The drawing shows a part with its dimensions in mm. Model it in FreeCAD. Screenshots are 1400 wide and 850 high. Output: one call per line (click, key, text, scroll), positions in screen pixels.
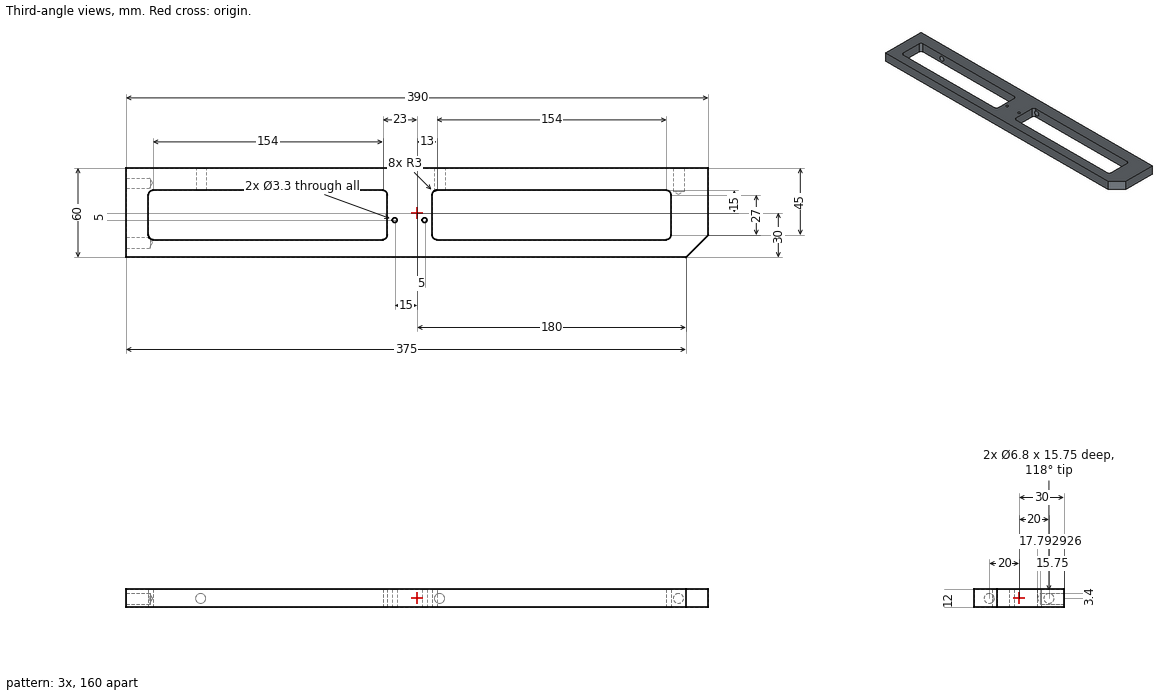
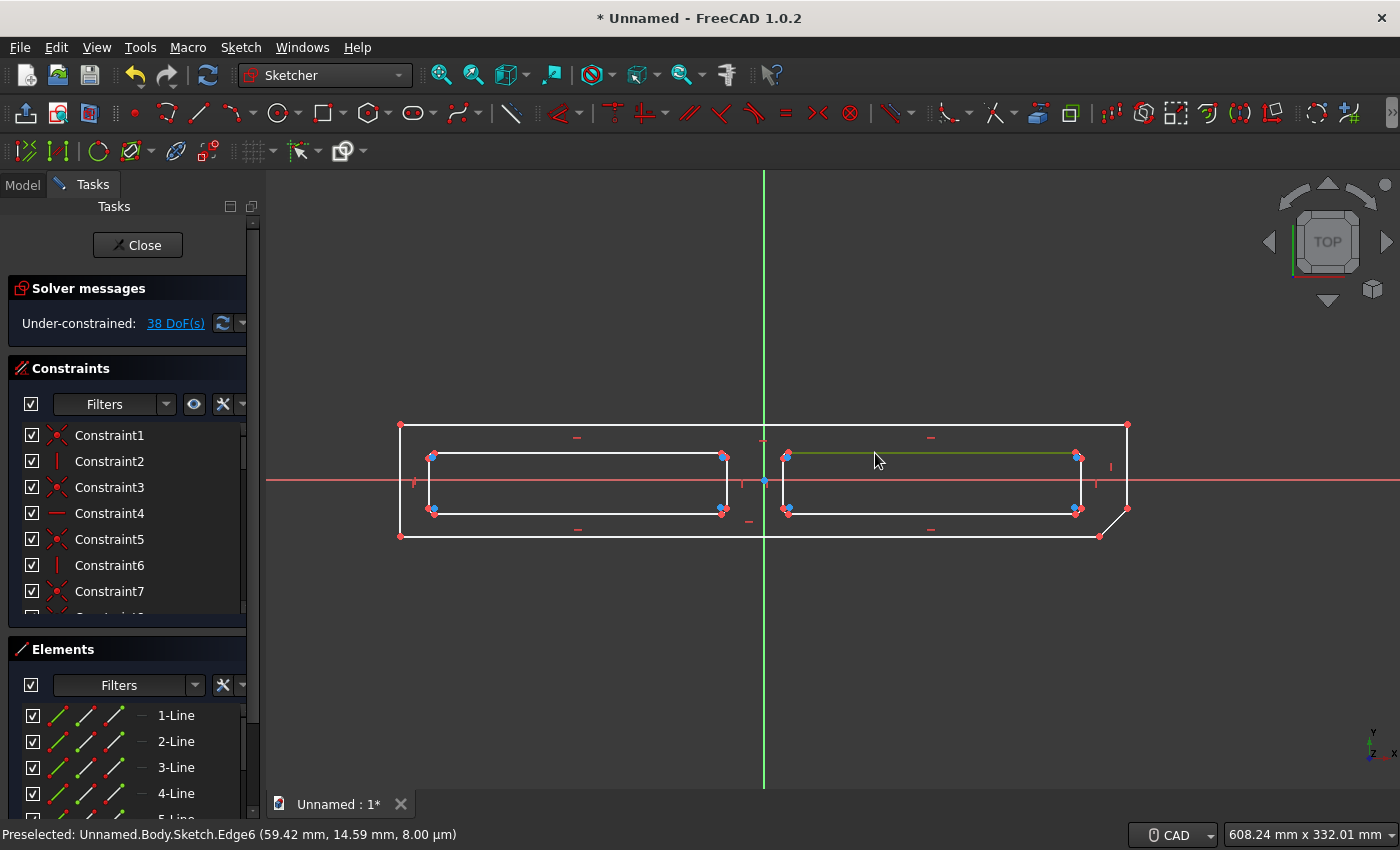
scroll(1080, 454, up, 6)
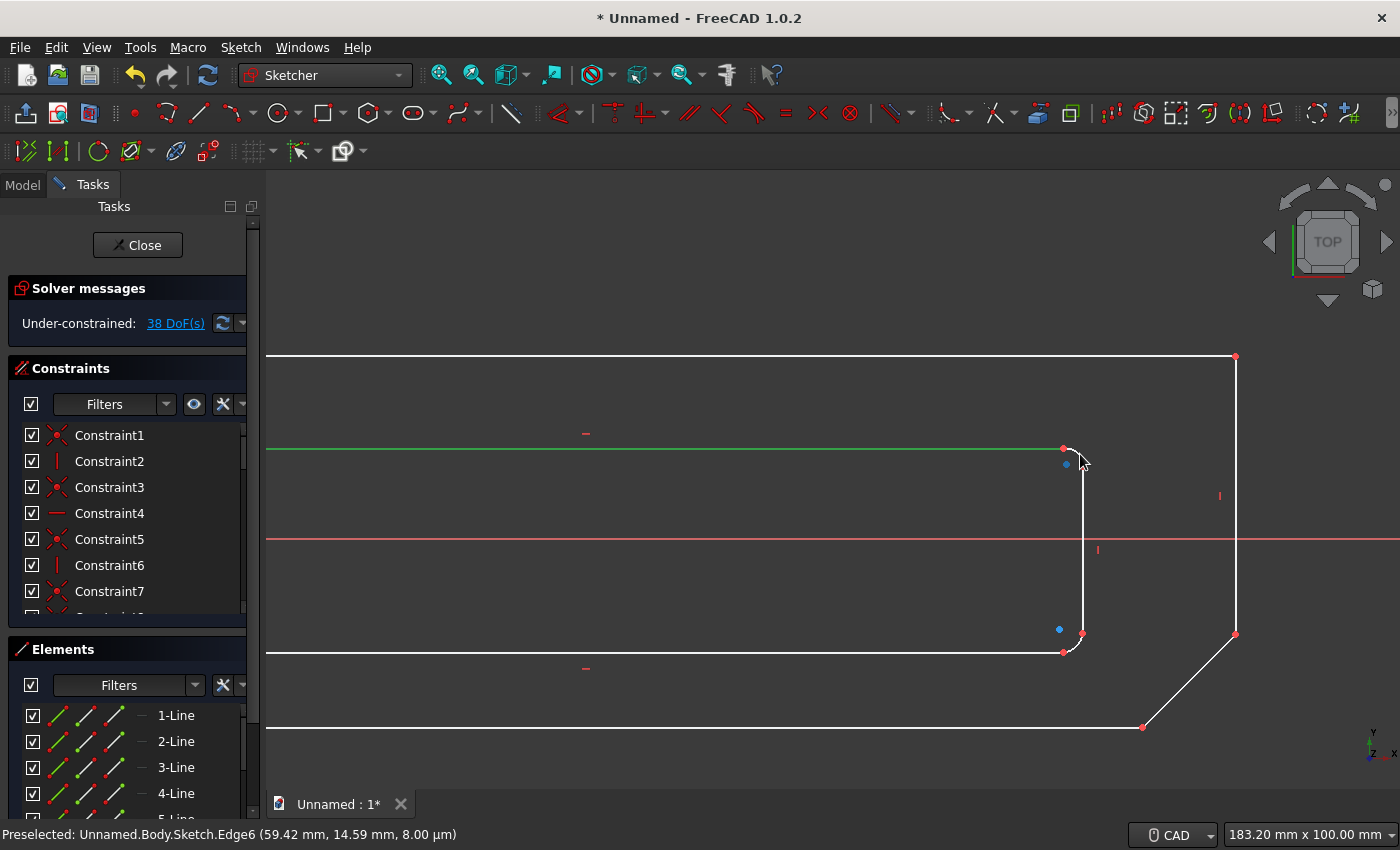
click(1077, 453)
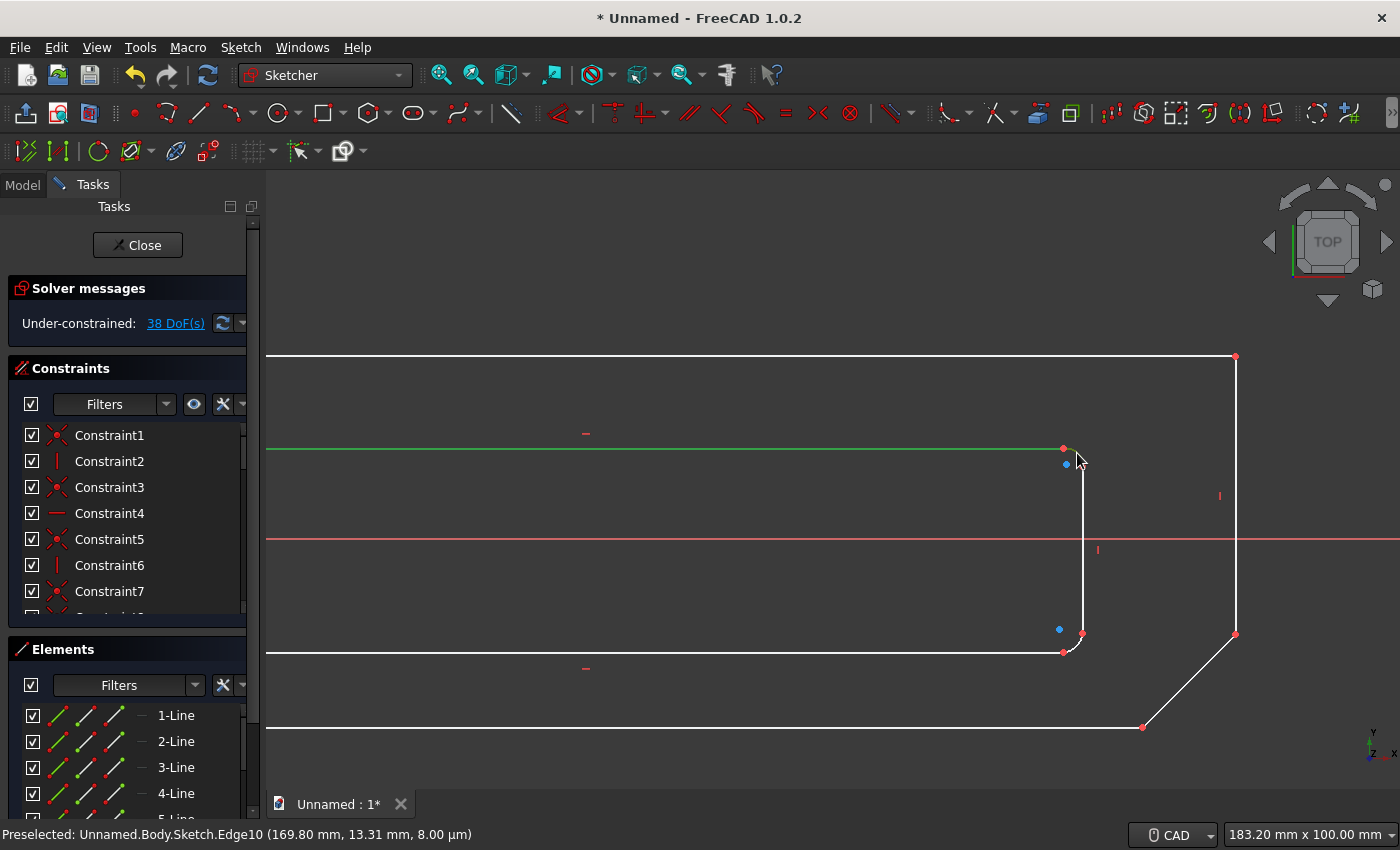
click(754, 114)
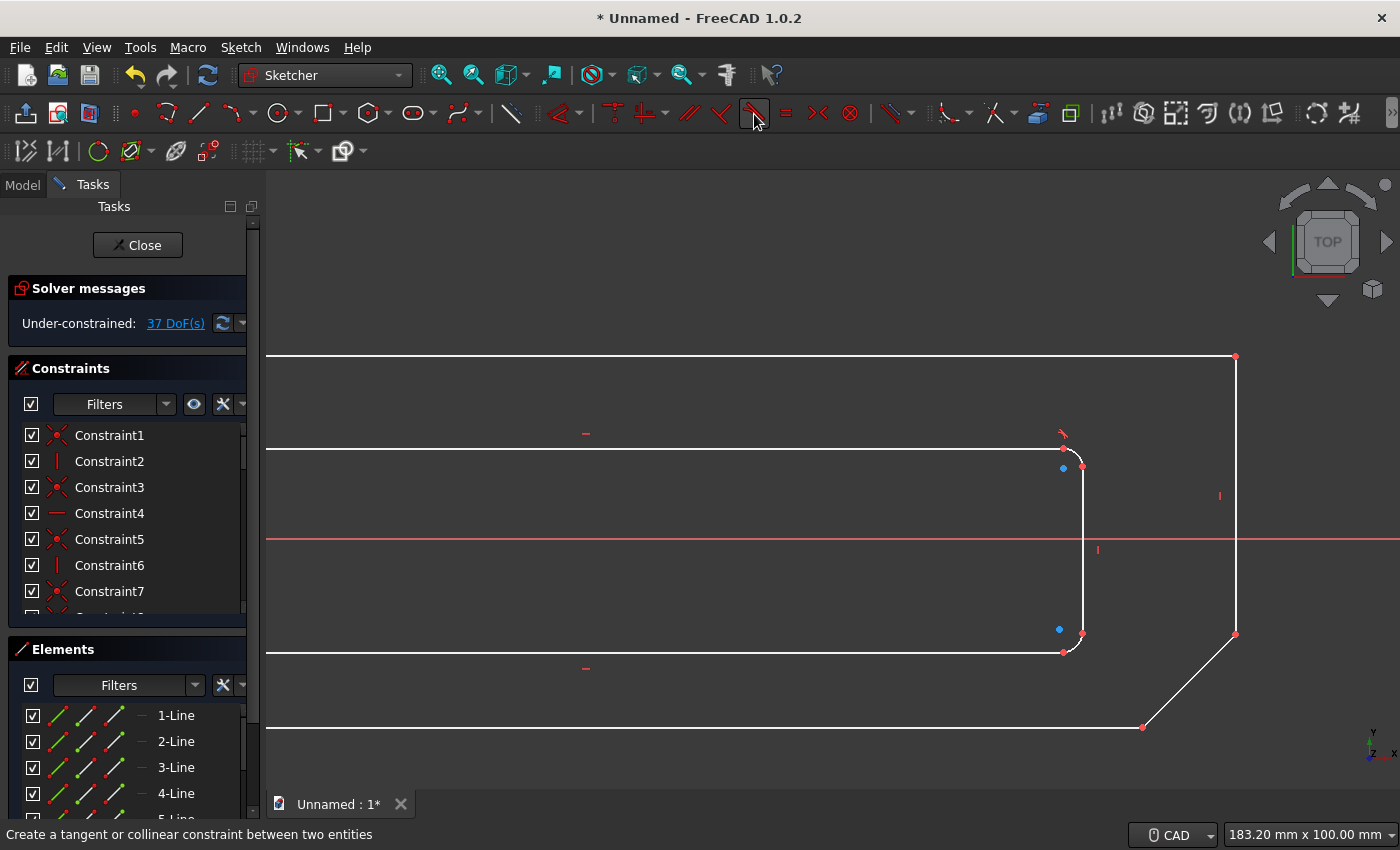
click(396, 449)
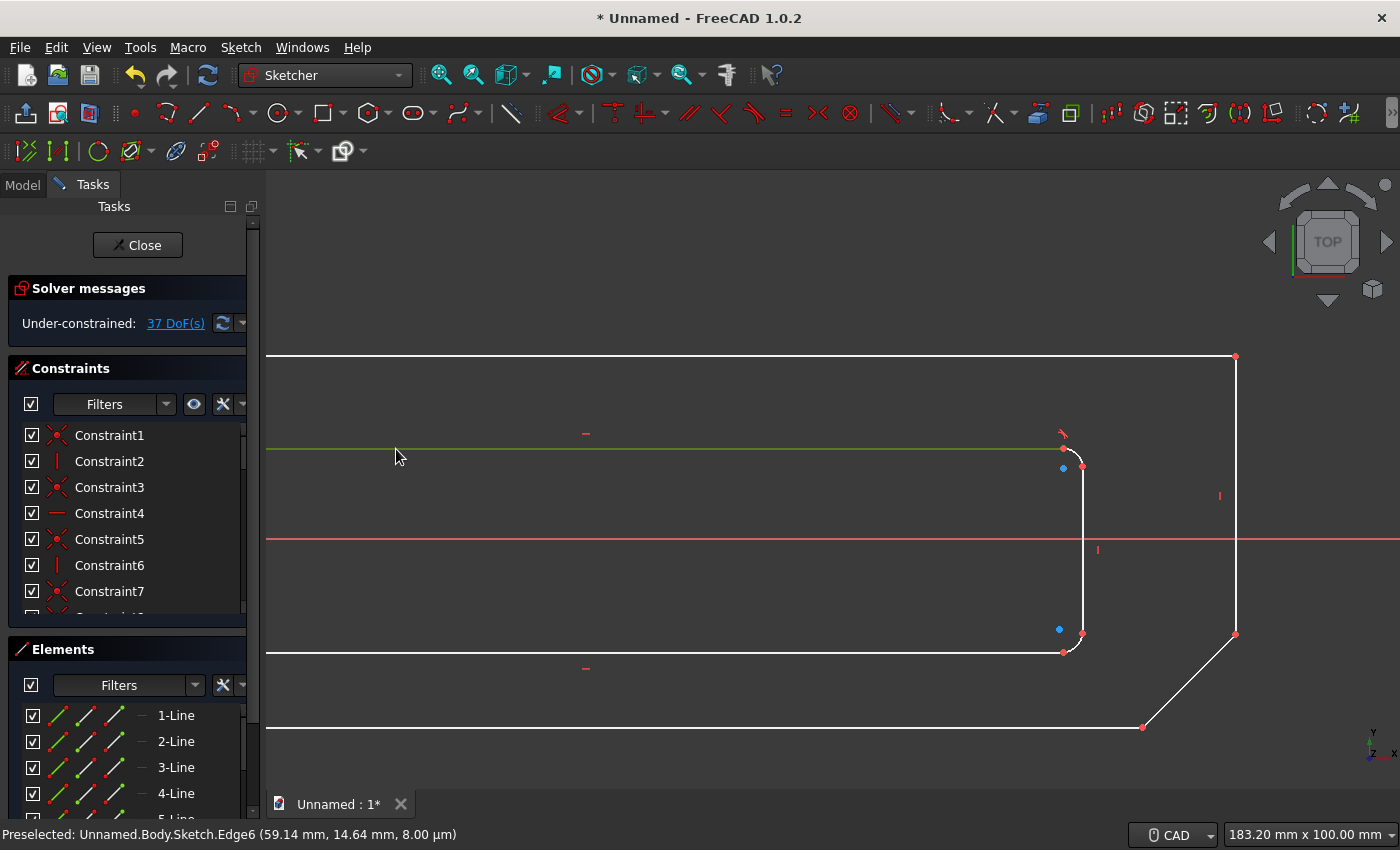
scroll(1081, 454, down, 6)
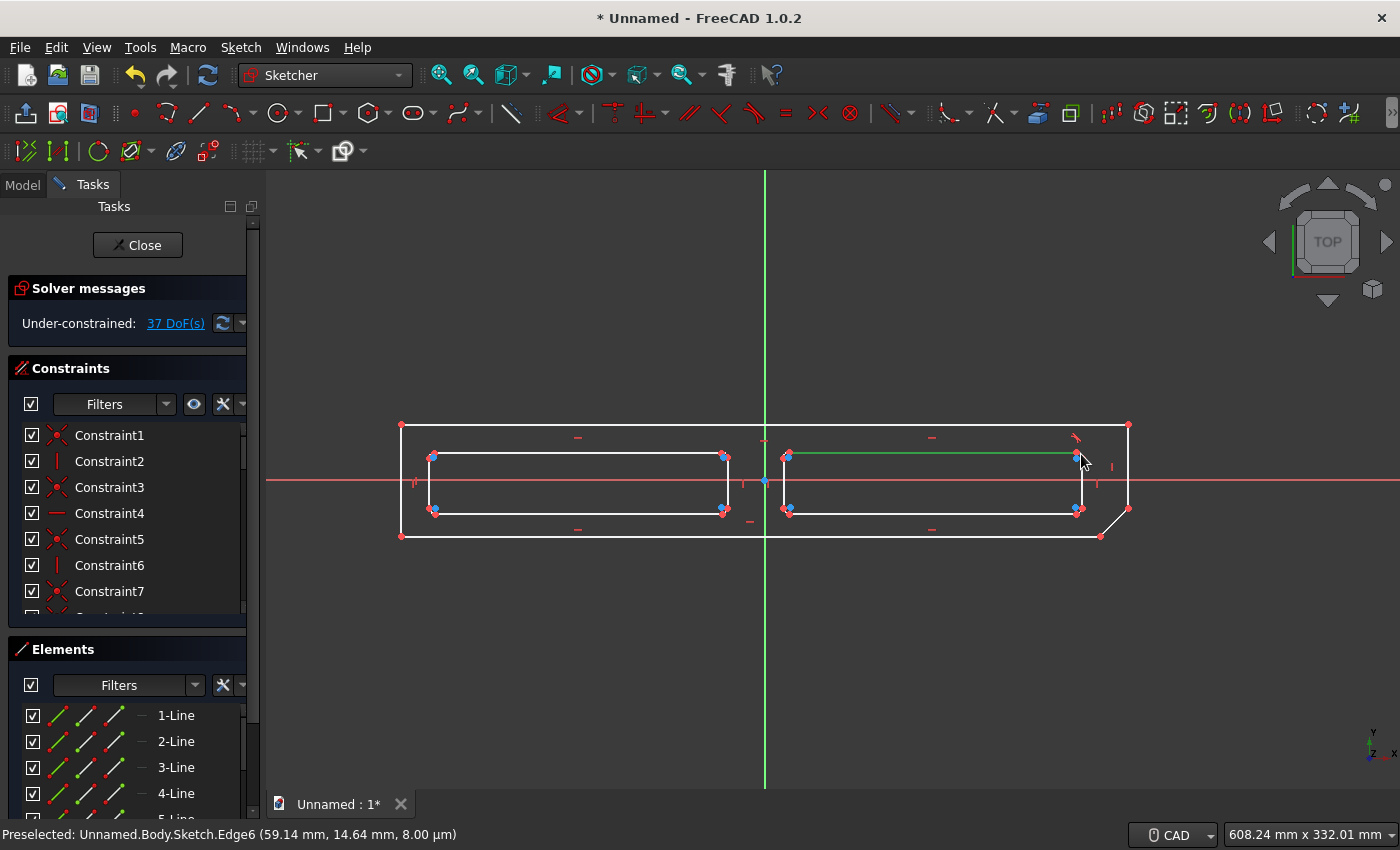
scroll(785, 454, up, 6)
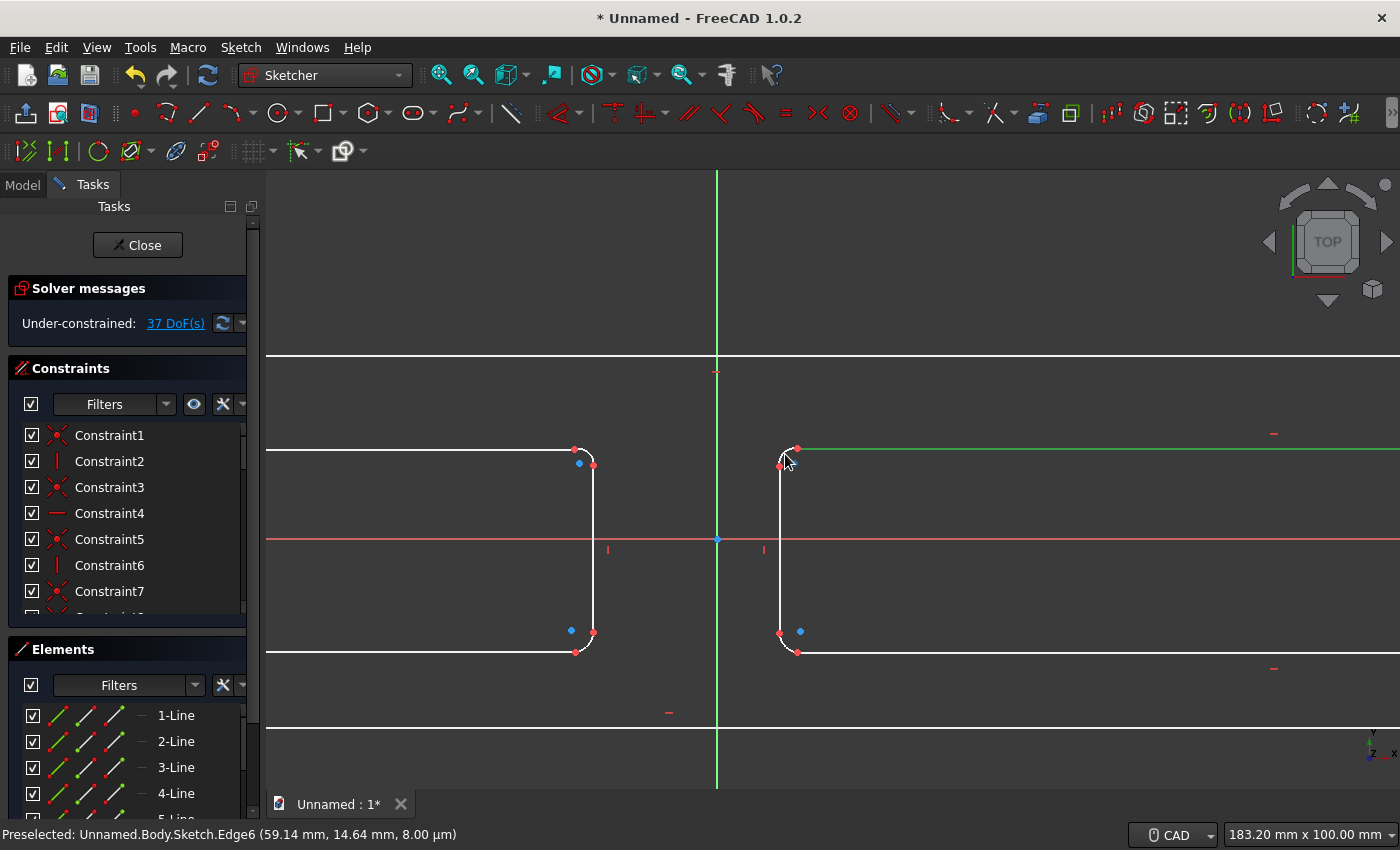
click(784, 453)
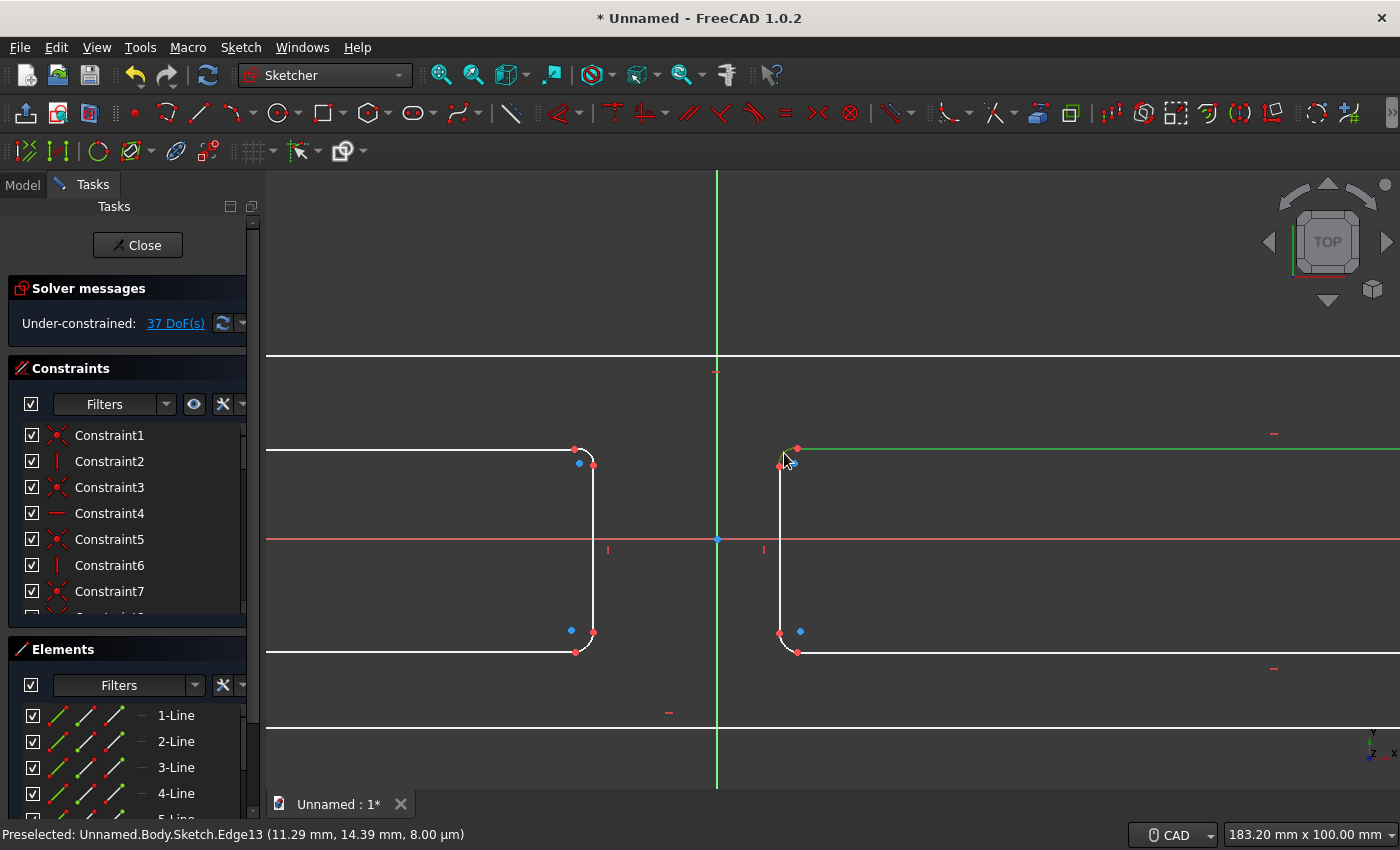
key(t)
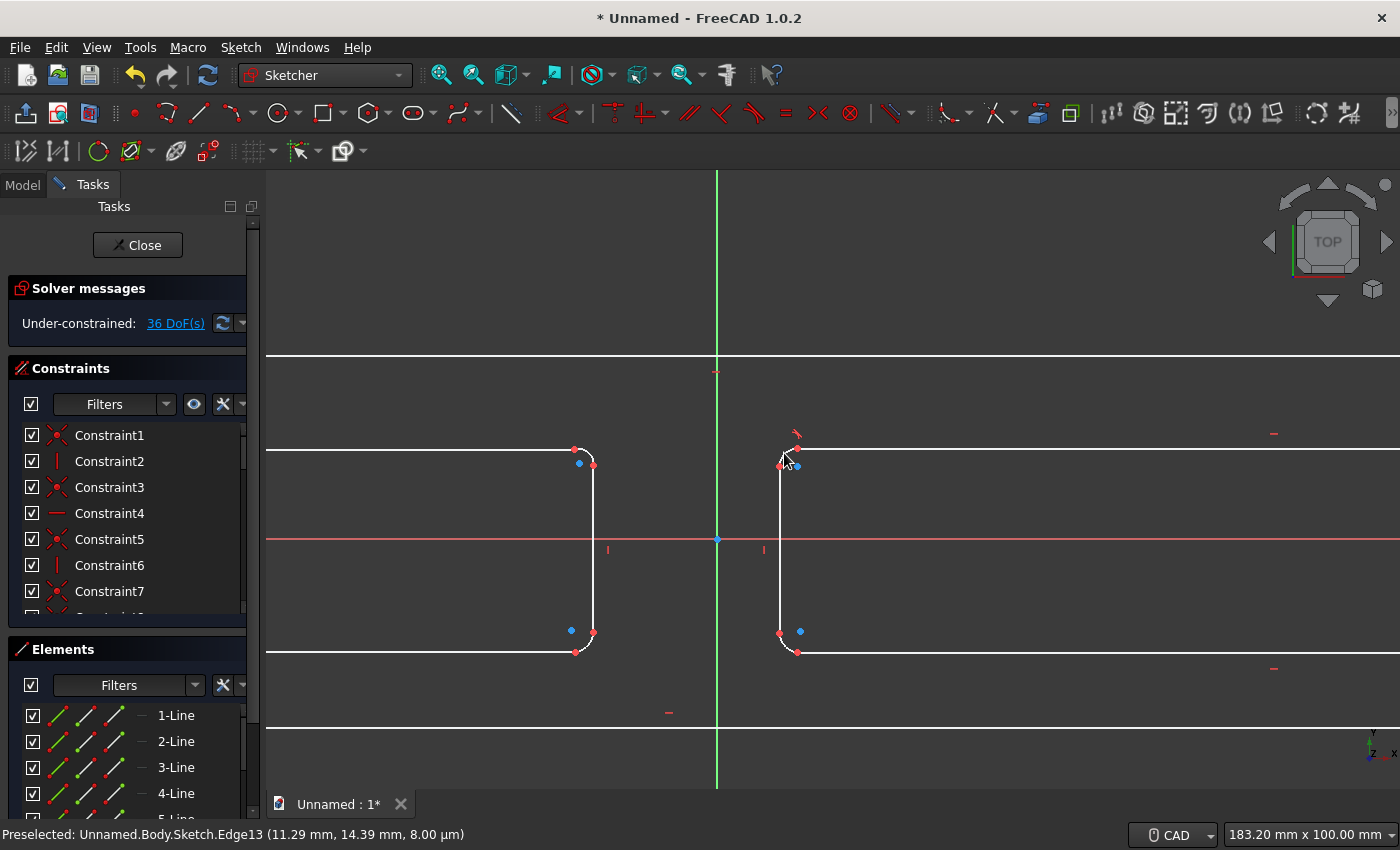
scroll(785, 454, down, 6)